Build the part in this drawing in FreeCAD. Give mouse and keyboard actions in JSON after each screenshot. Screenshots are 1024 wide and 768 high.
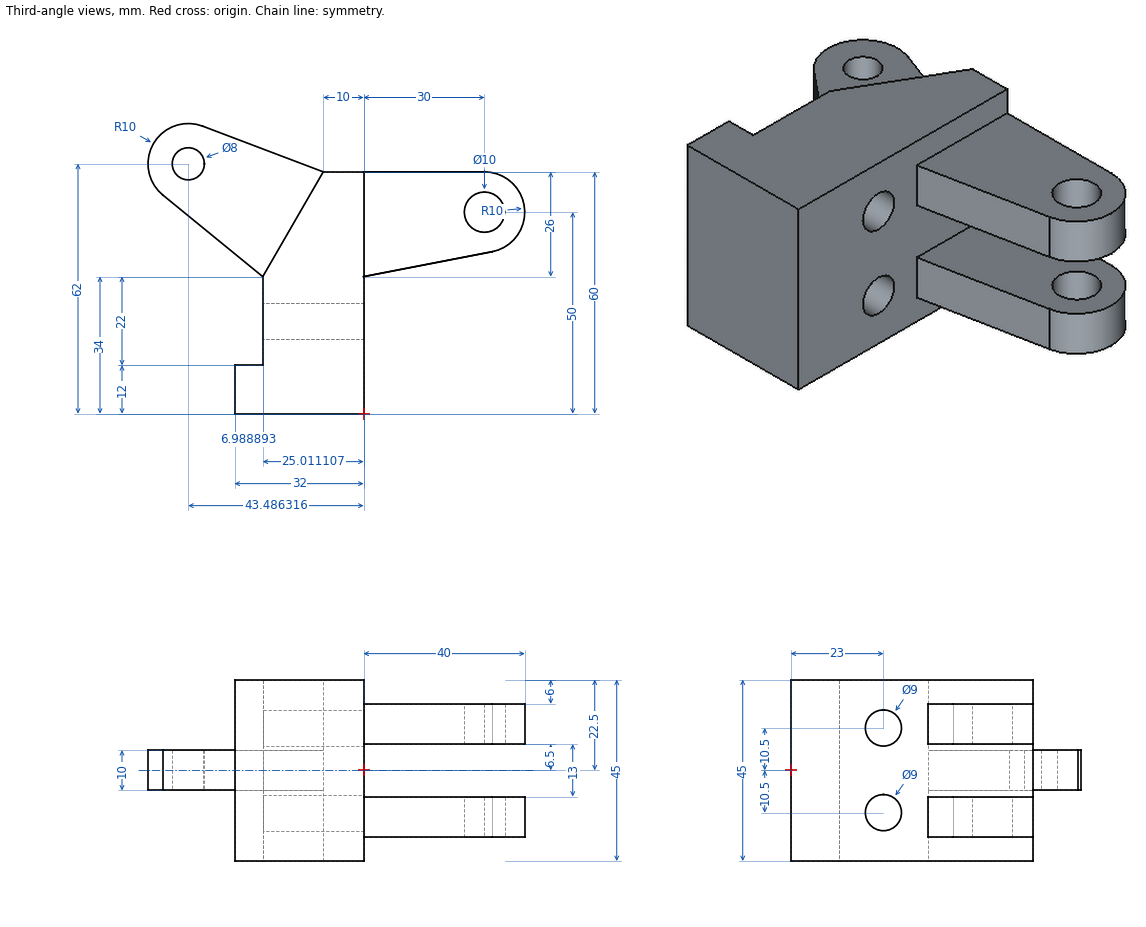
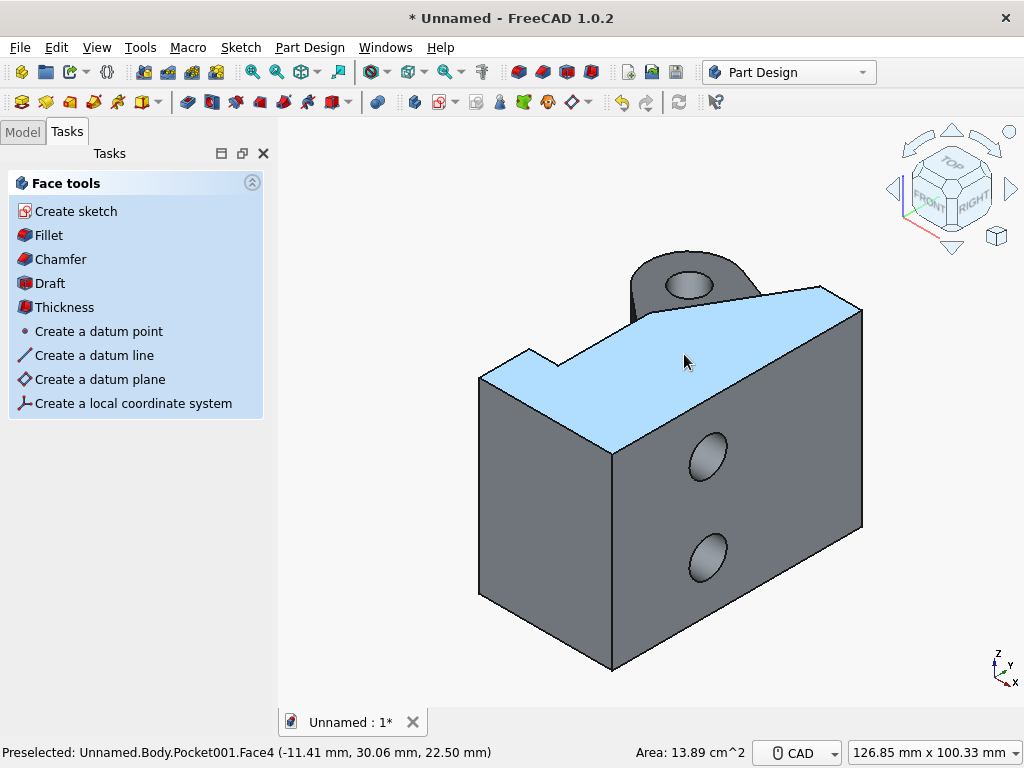
{"action": "left_click", "coordinate": [440, 102]}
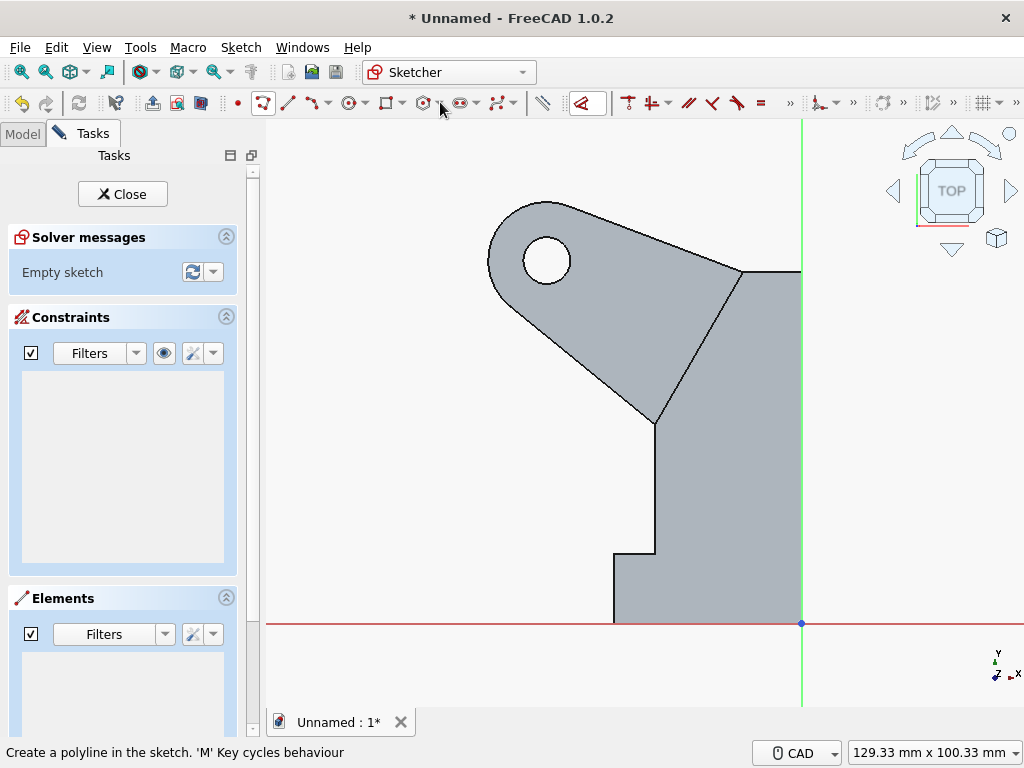
{"action": "scroll", "coordinate": [294, 342], "scroll_direction": "down", "scroll_amount": 2}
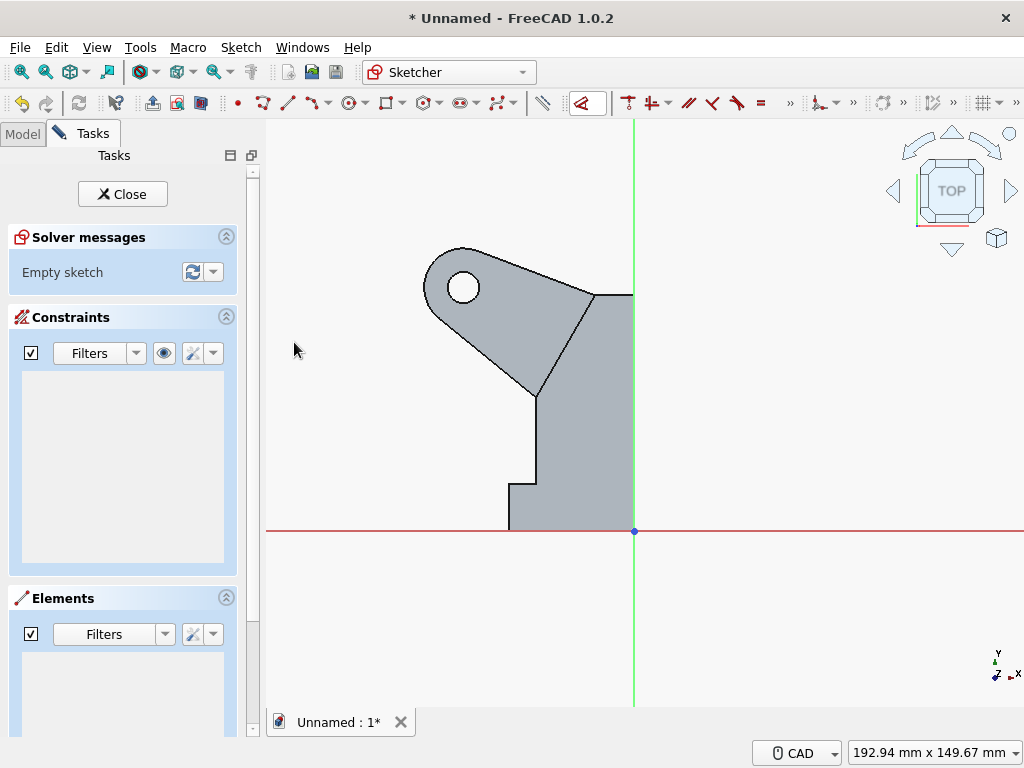
{"action": "scroll", "coordinate": [859, 414], "scroll_direction": "up", "scroll_amount": 2}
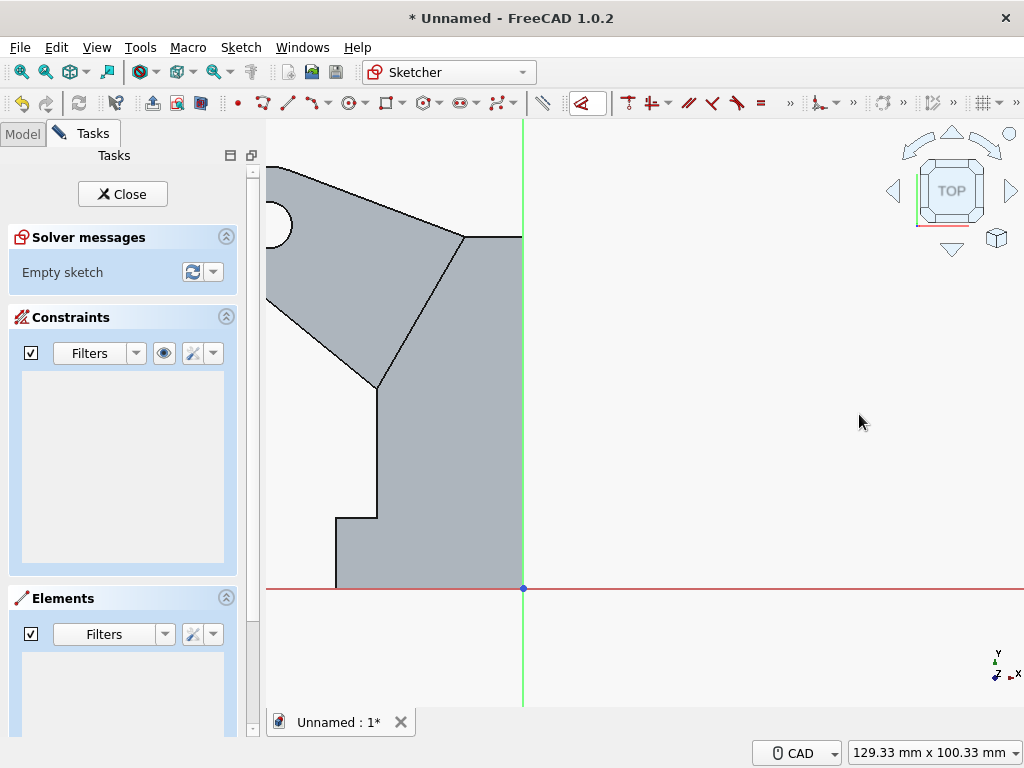
{"action": "key", "text": "g m"}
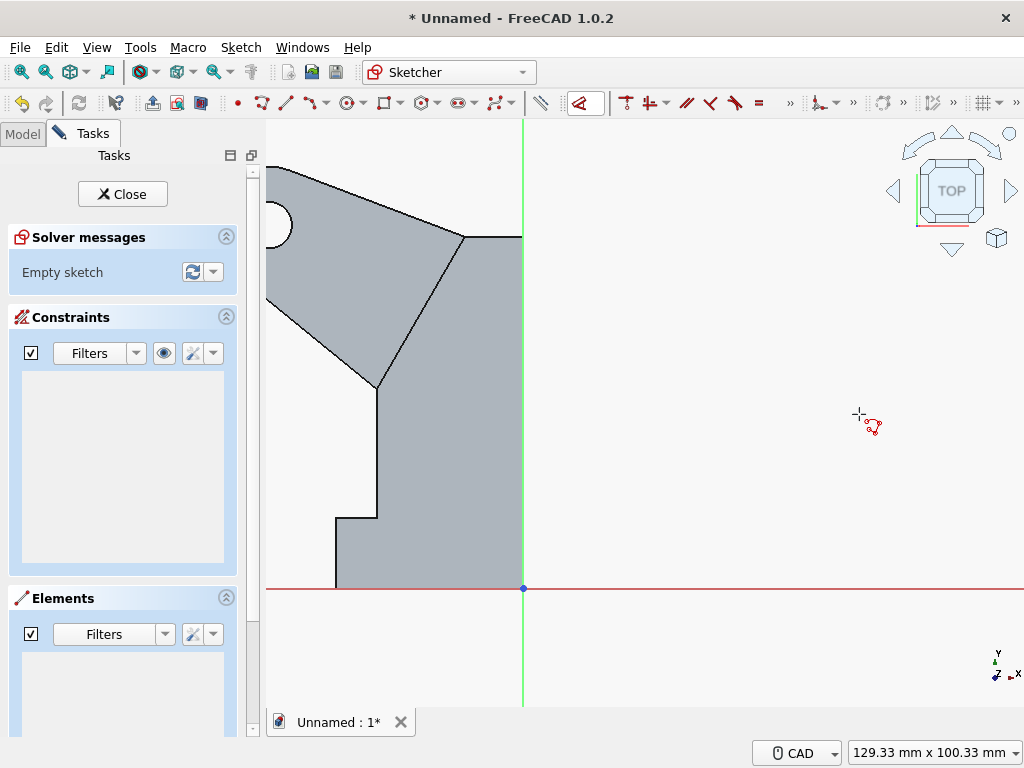
{"action": "left_click", "coordinate": [699, 237]}
{"action": "left_click", "coordinate": [523, 237]}
{"action": "left_click", "coordinate": [532, 389]}
{"action": "left_click", "coordinate": [710, 353]}
{"action": "right_click", "coordinate": [710, 353]}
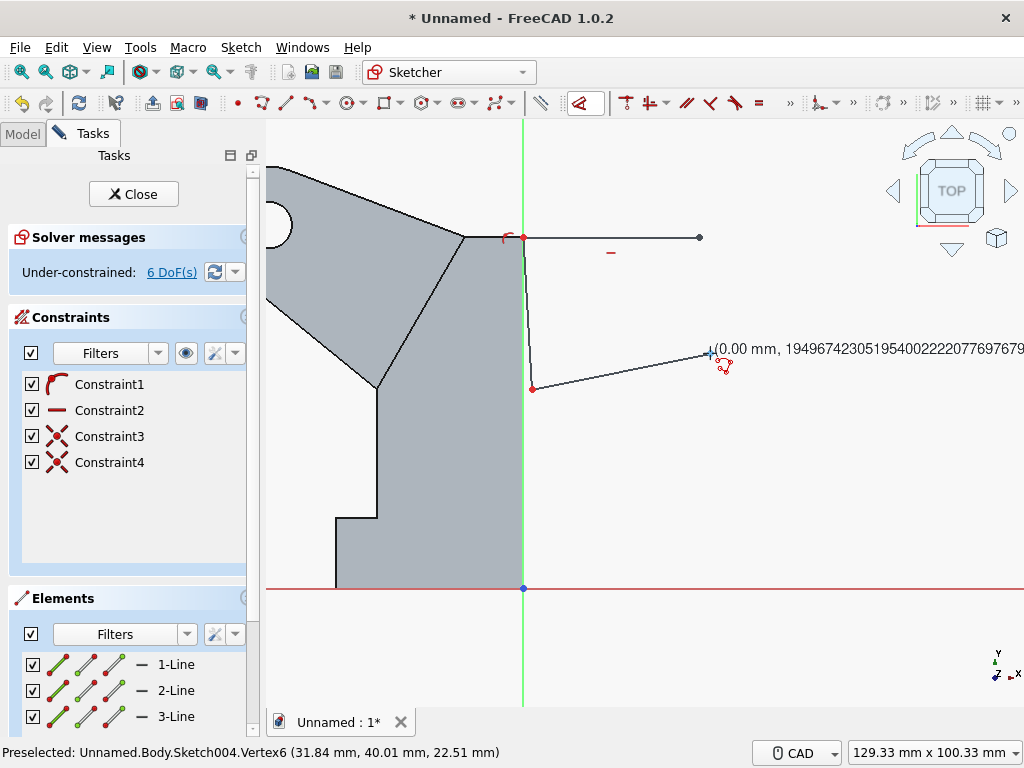
{"action": "key", "text": "g 3 a"}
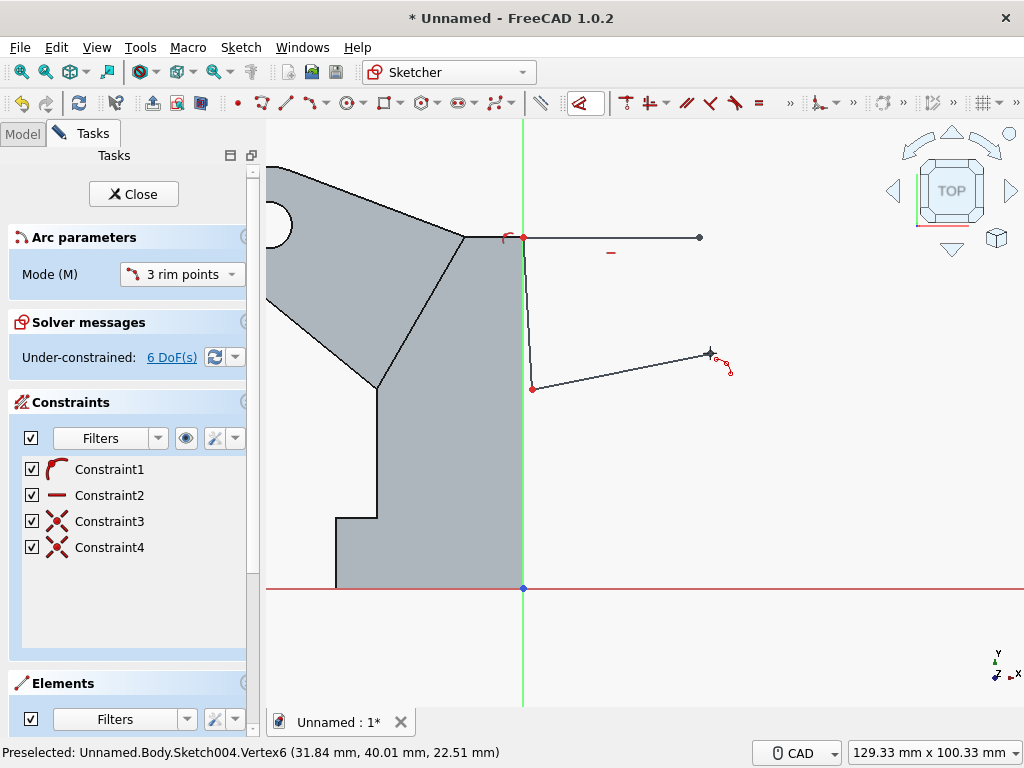
{"action": "left_click", "coordinate": [710, 354]}
{"action": "left_click", "coordinate": [699, 238]}
{"action": "left_click", "coordinate": [758, 290]}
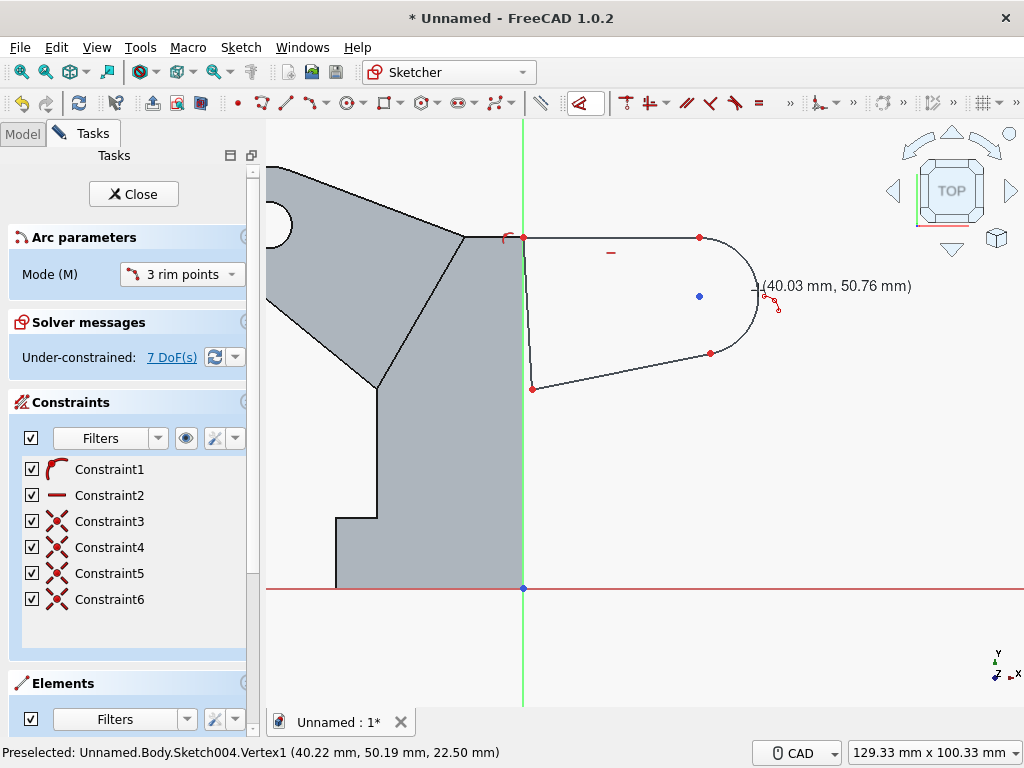
{"action": "left_click", "coordinate": [348, 104]}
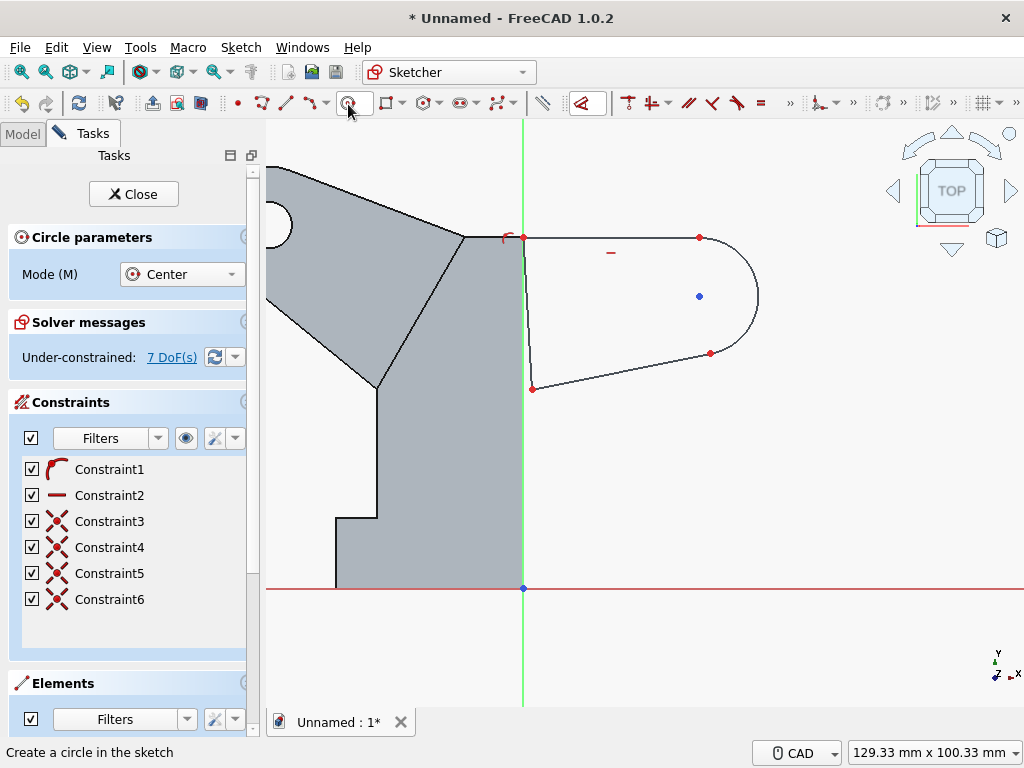
{"action": "left_click", "coordinate": [699, 295]}
{"action": "mouse_move", "coordinate": [720, 275]}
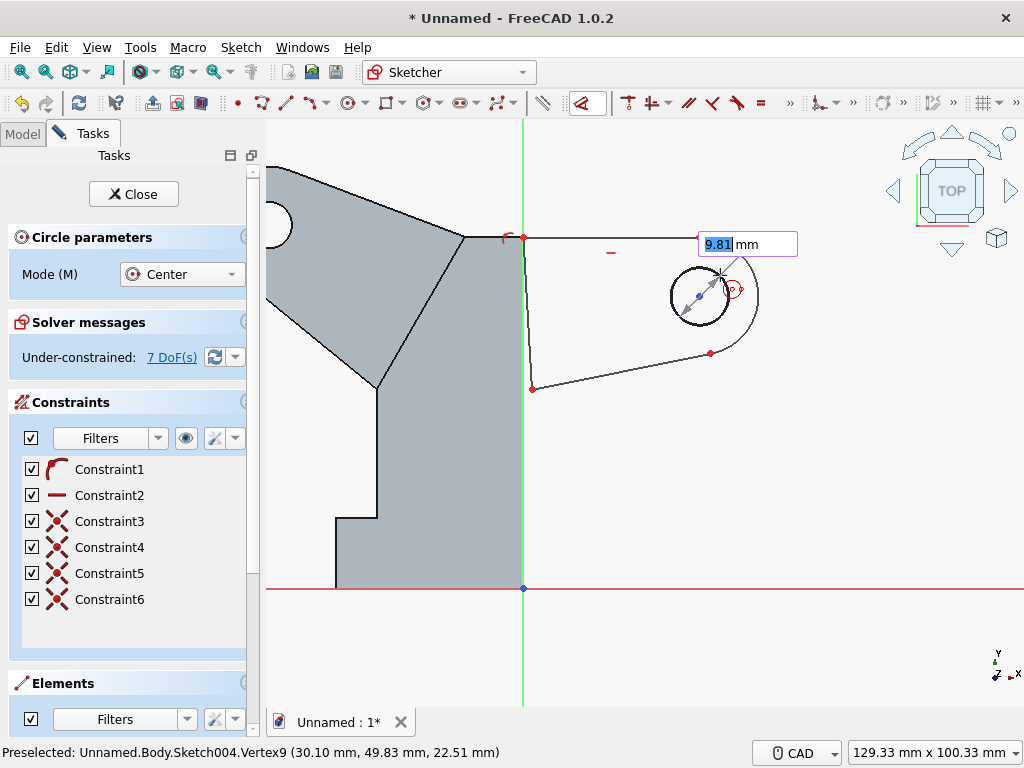
{"action": "type", "text": "10"}
{"action": "key", "text": "Return"}
{"action": "key", "text": "Escape"}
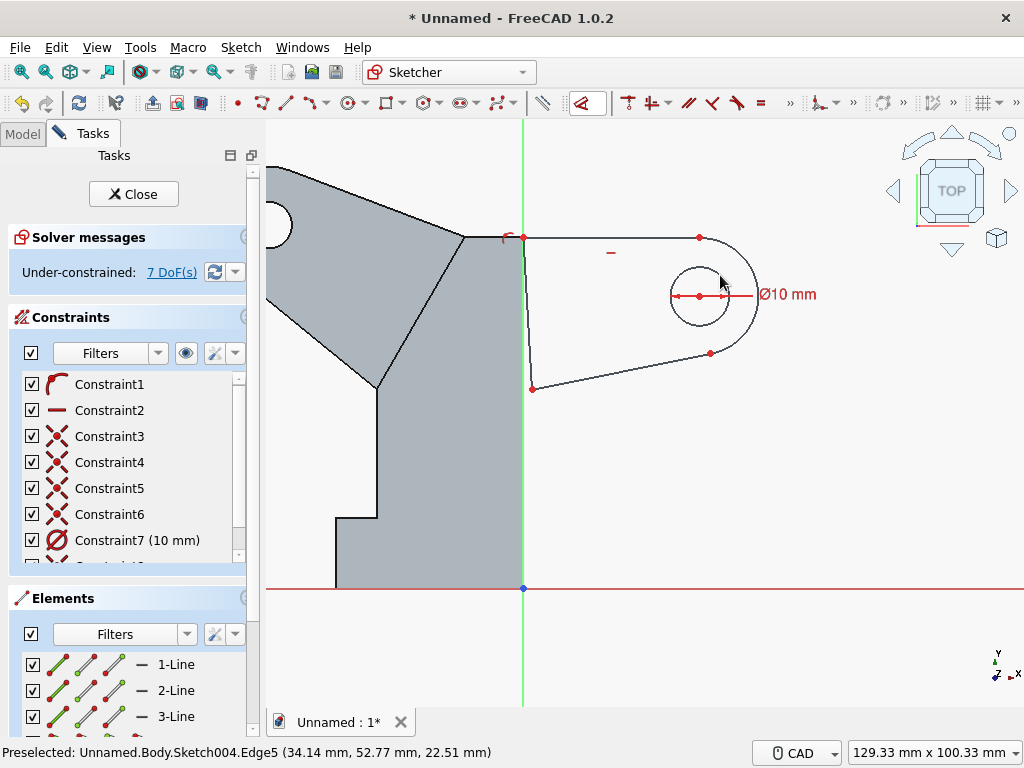
{"action": "left_click", "coordinate": [646, 238]}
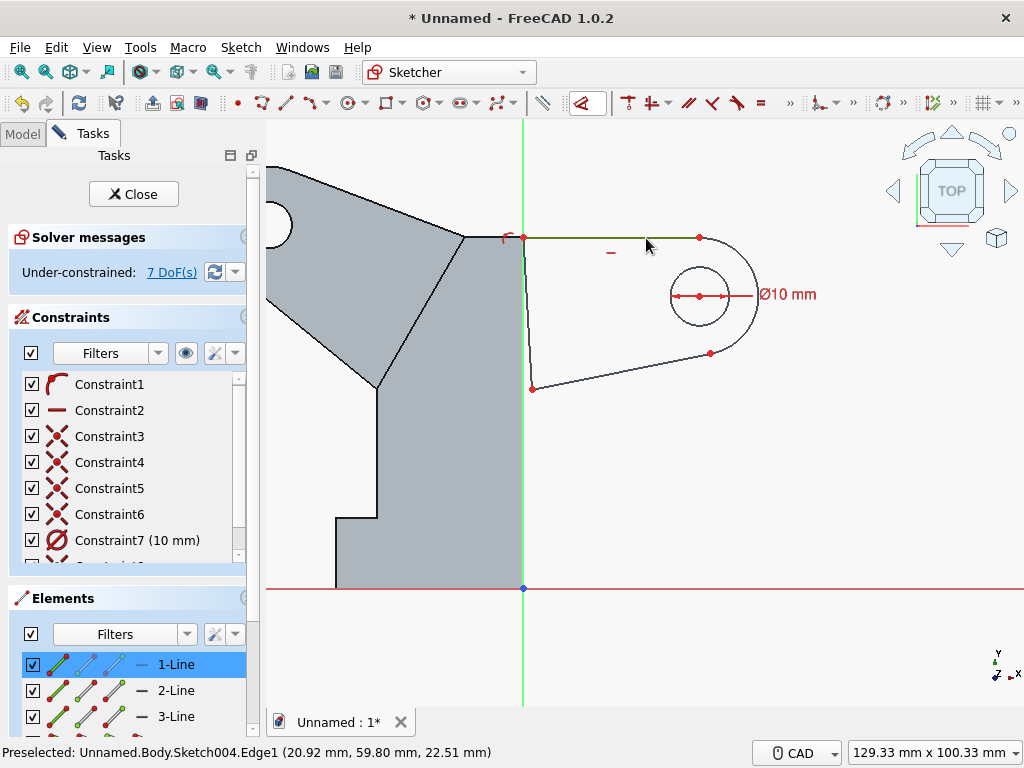
{"action": "left_click", "coordinate": [751, 325]}